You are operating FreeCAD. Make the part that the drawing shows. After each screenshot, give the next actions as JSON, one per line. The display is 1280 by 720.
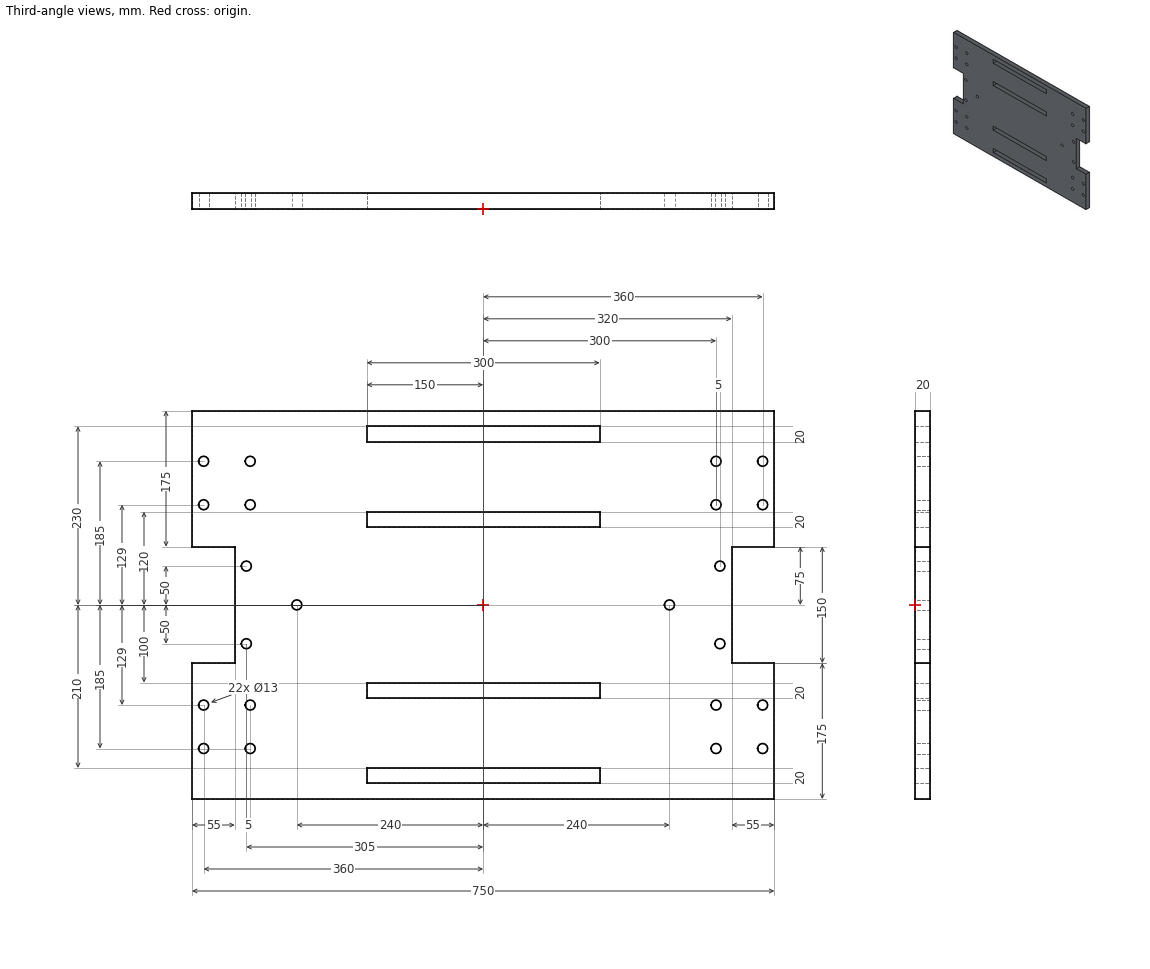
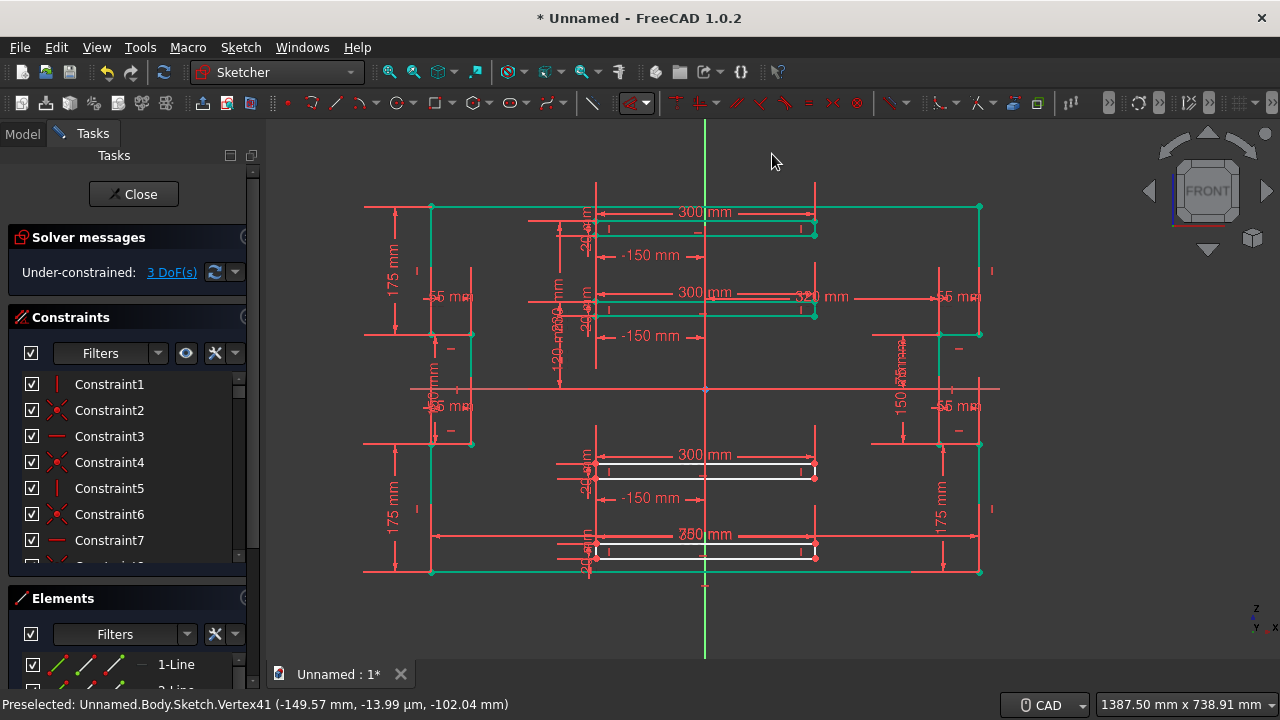
{"action": "left_click", "coordinate": [596, 464]}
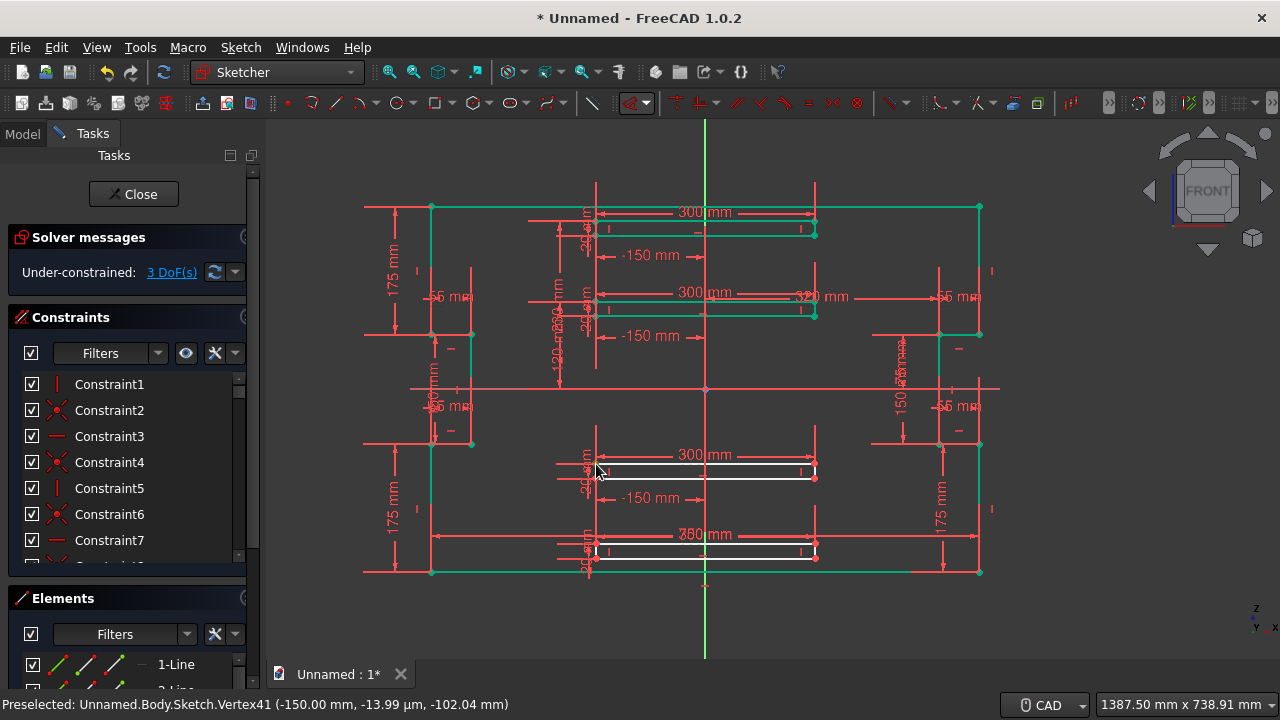
{"action": "key", "text": "i"}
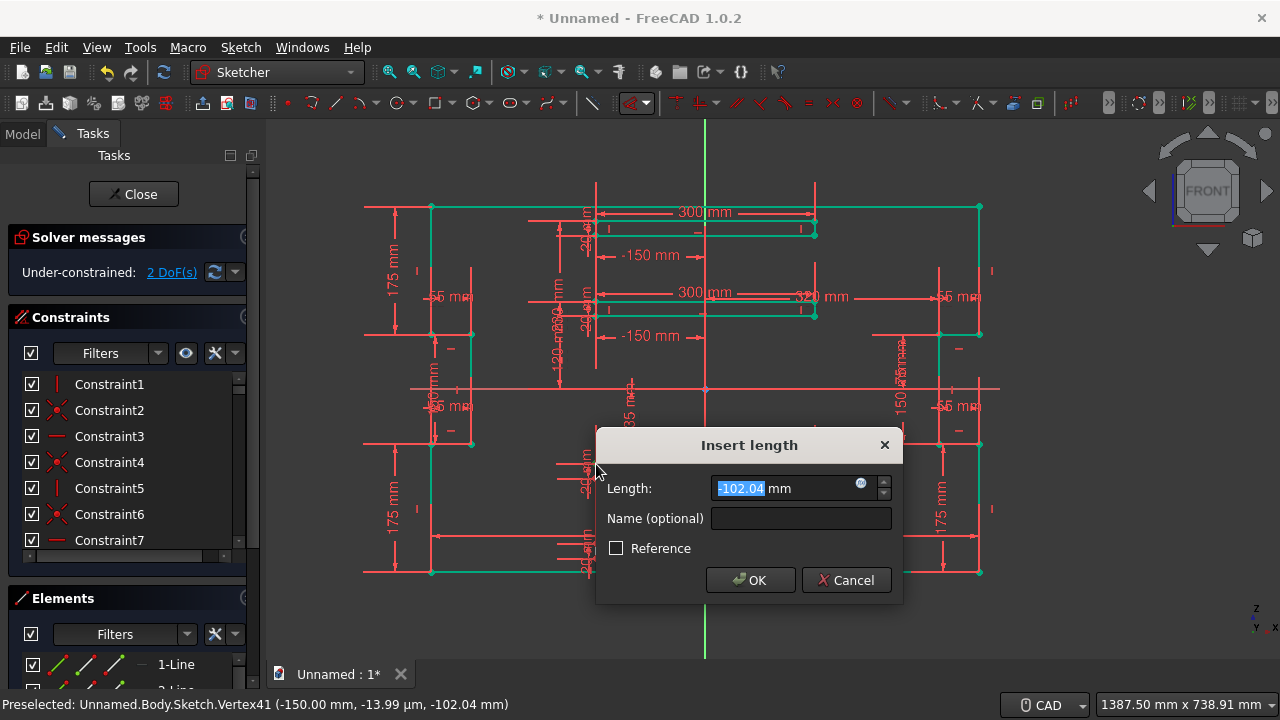
{"action": "type", "text": "-100"}
{"action": "key", "text": "Return"}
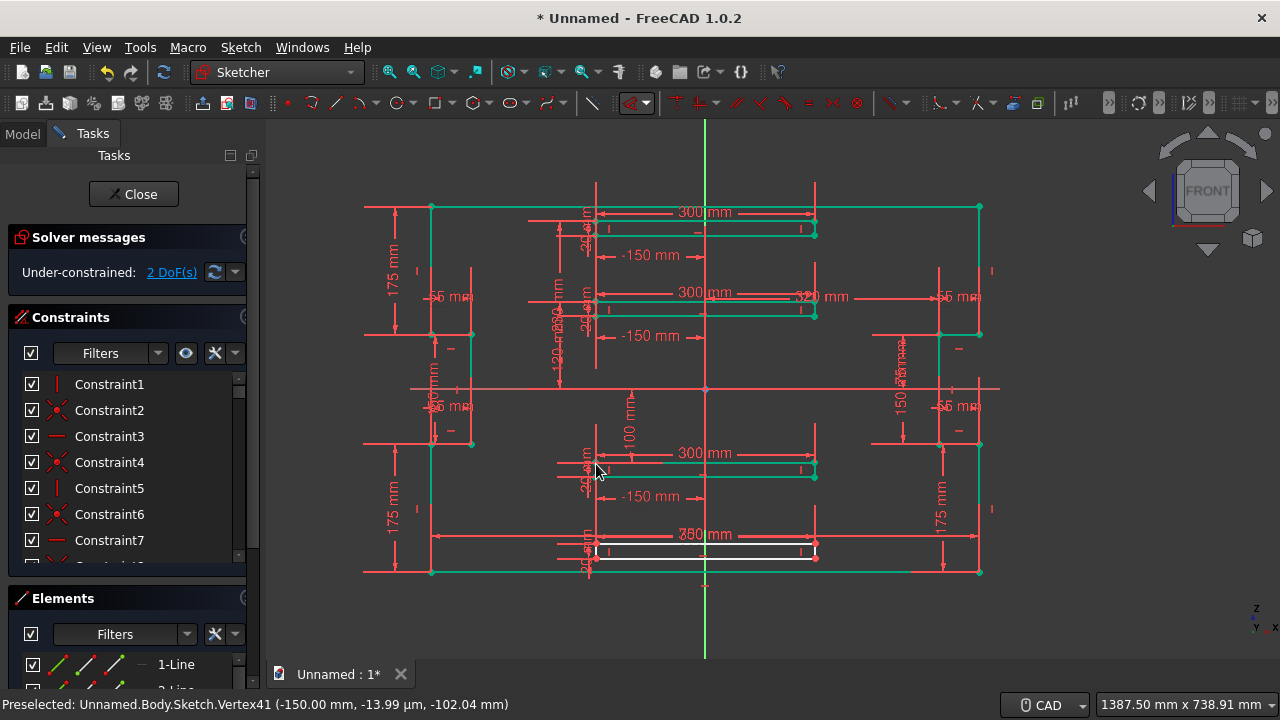
{"action": "left_click", "coordinate": [596, 544]}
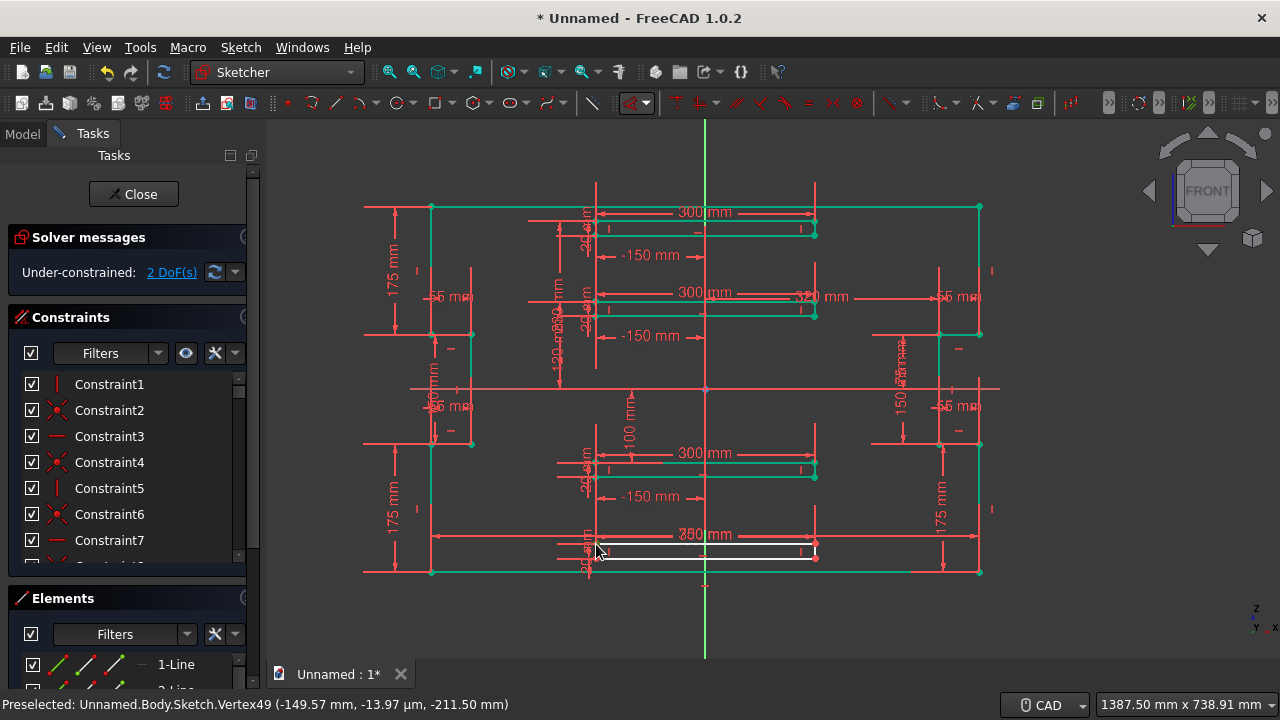
{"action": "left_click", "coordinate": [648, 104]}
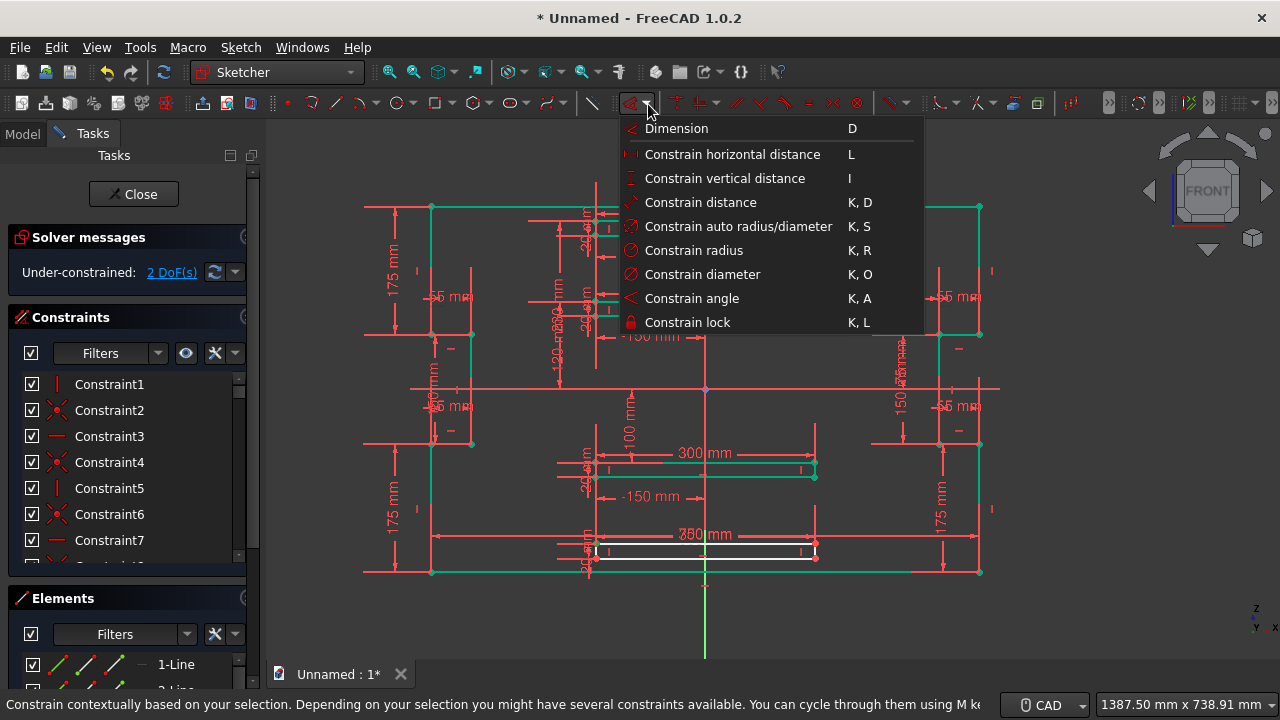
{"action": "left_click", "coordinate": [772, 154]}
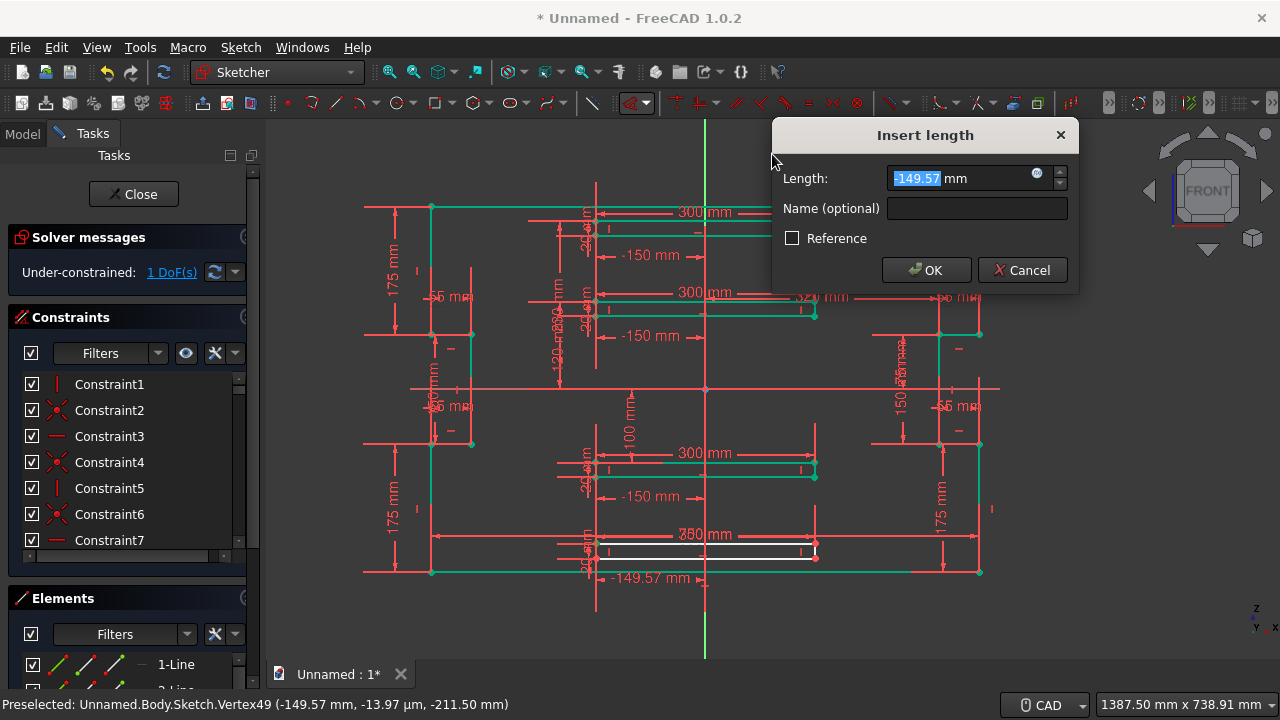
{"action": "type", "text": "-150"}
{"action": "key", "text": "Return"}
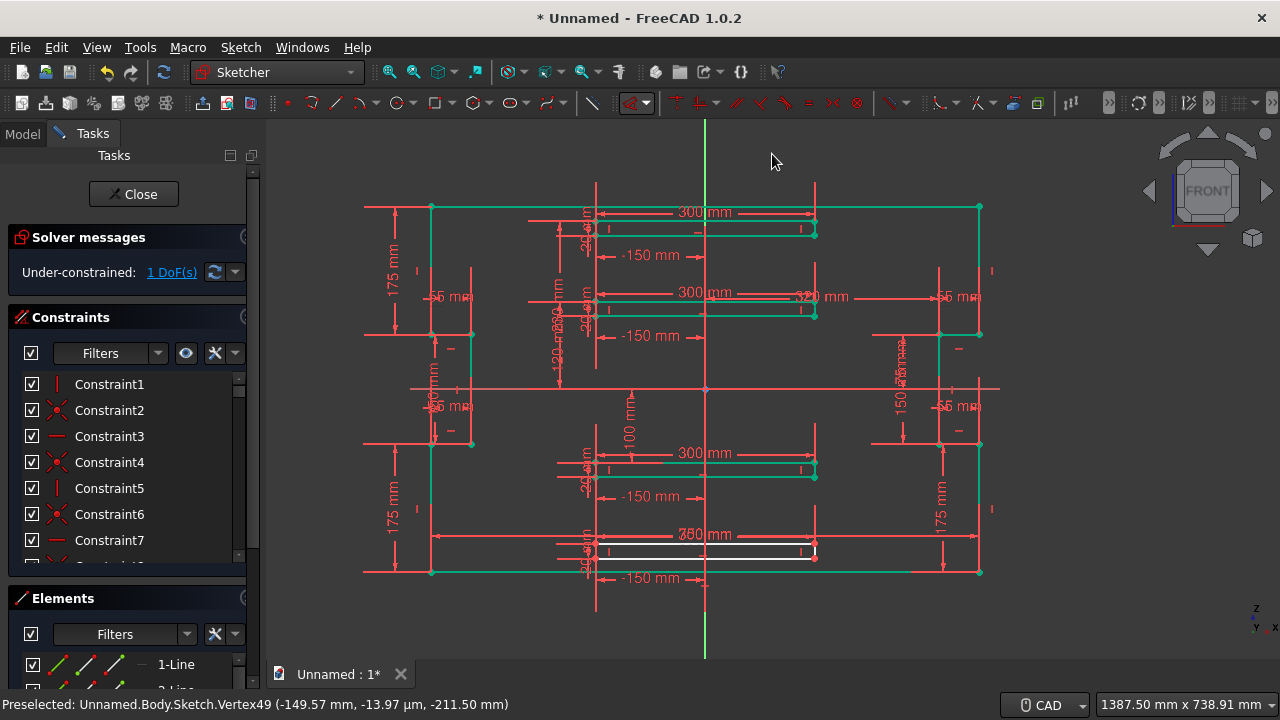
{"action": "left_click", "coordinate": [596, 544]}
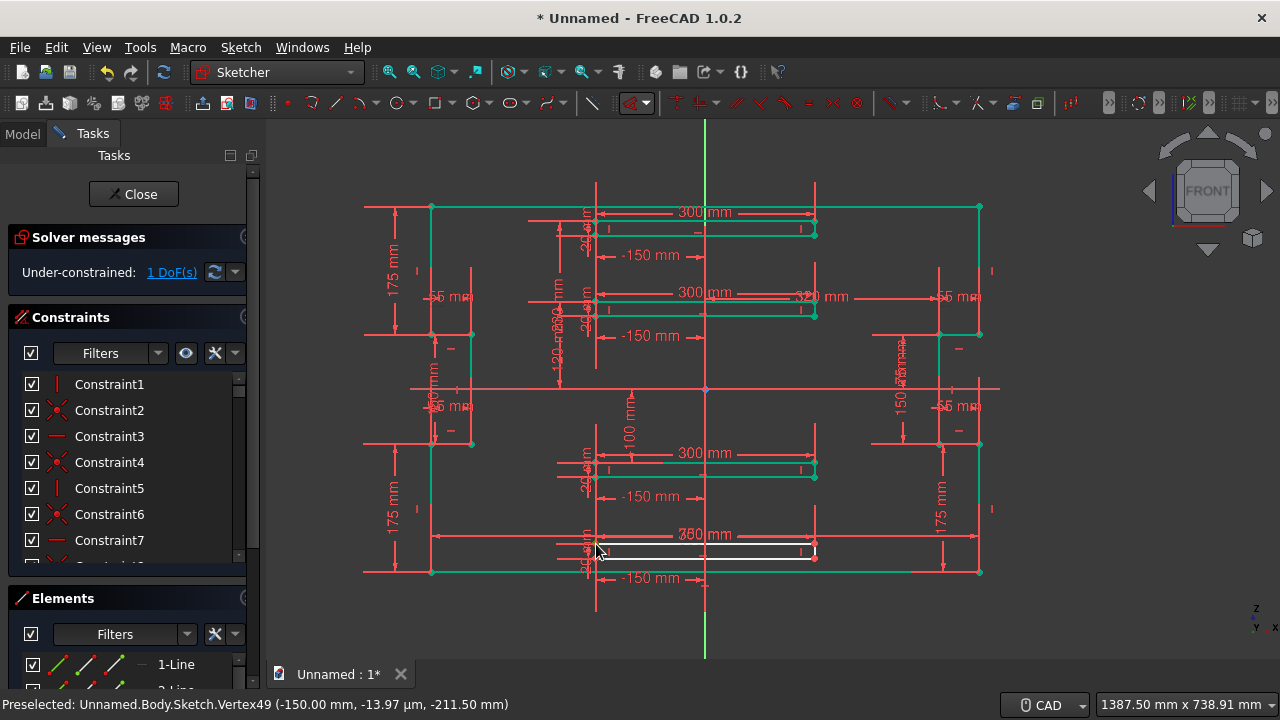
{"action": "key", "text": "i"}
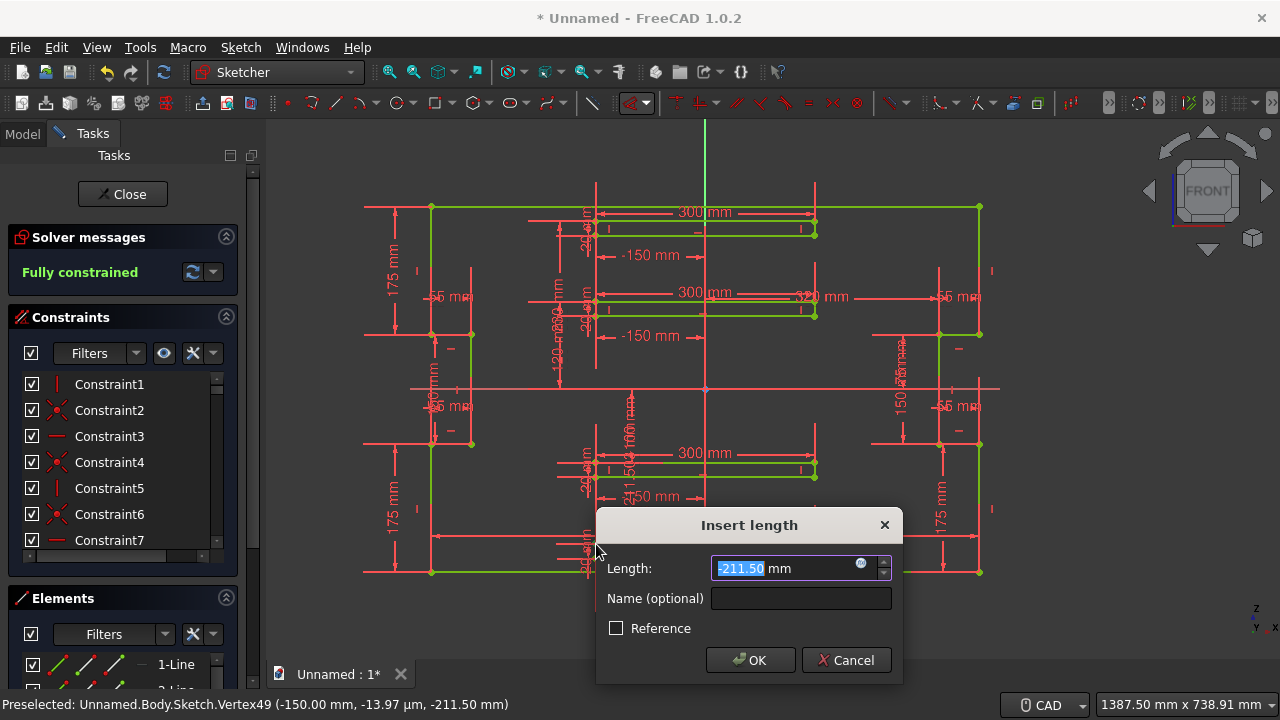
{"action": "type", "text": "-210"}
{"action": "key", "text": "Return"}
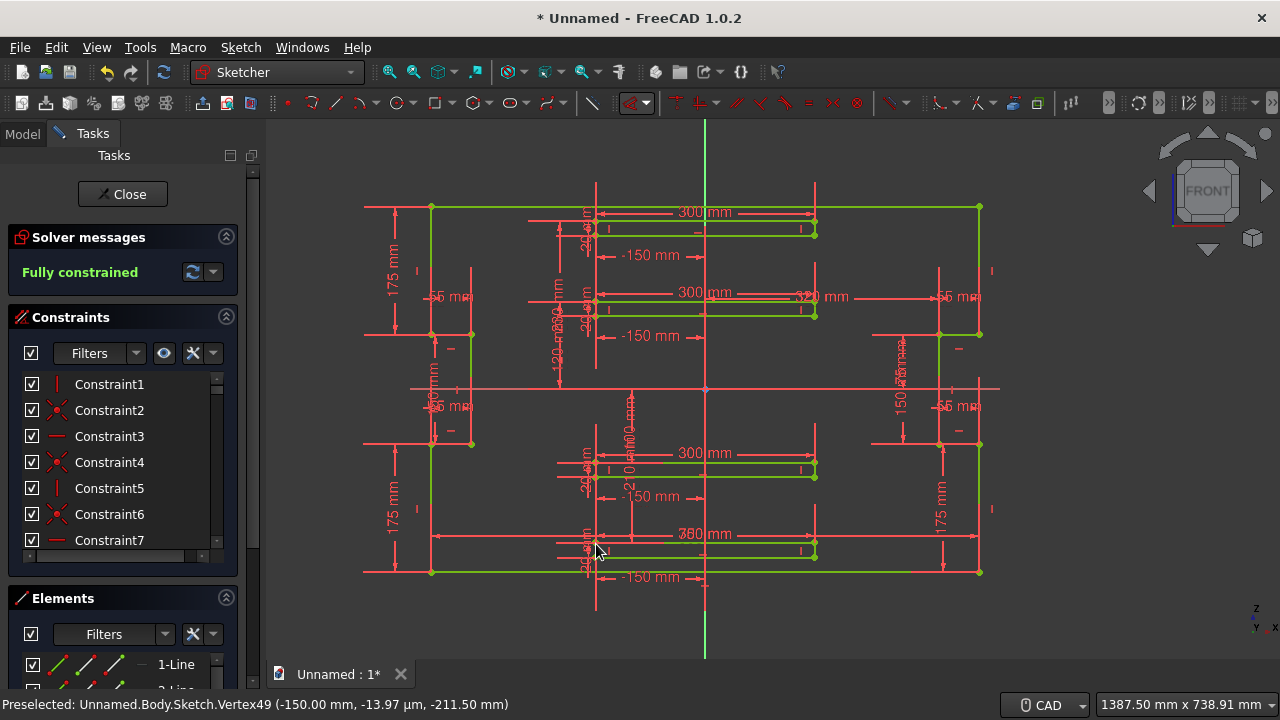
{"action": "left_click", "coordinate": [123, 194]}